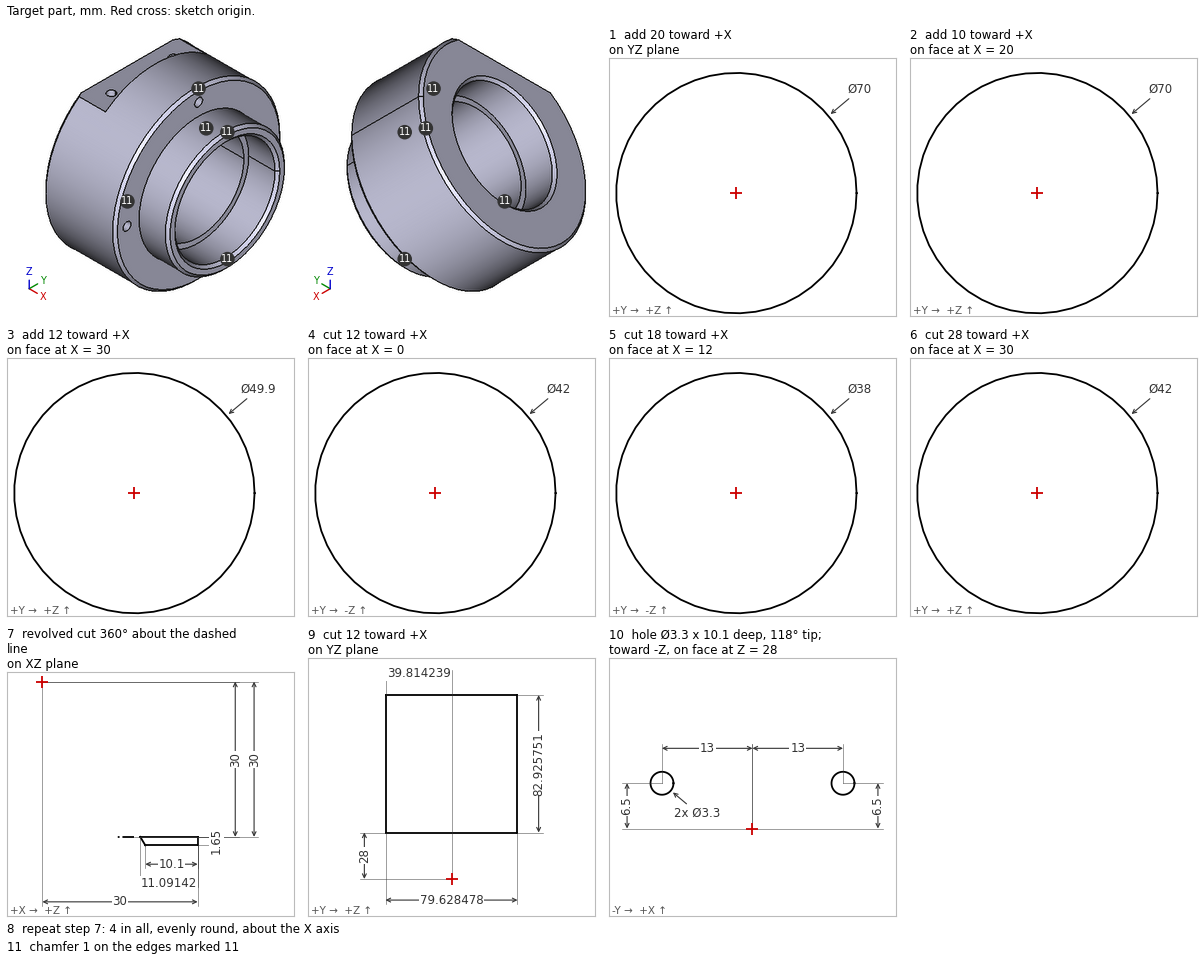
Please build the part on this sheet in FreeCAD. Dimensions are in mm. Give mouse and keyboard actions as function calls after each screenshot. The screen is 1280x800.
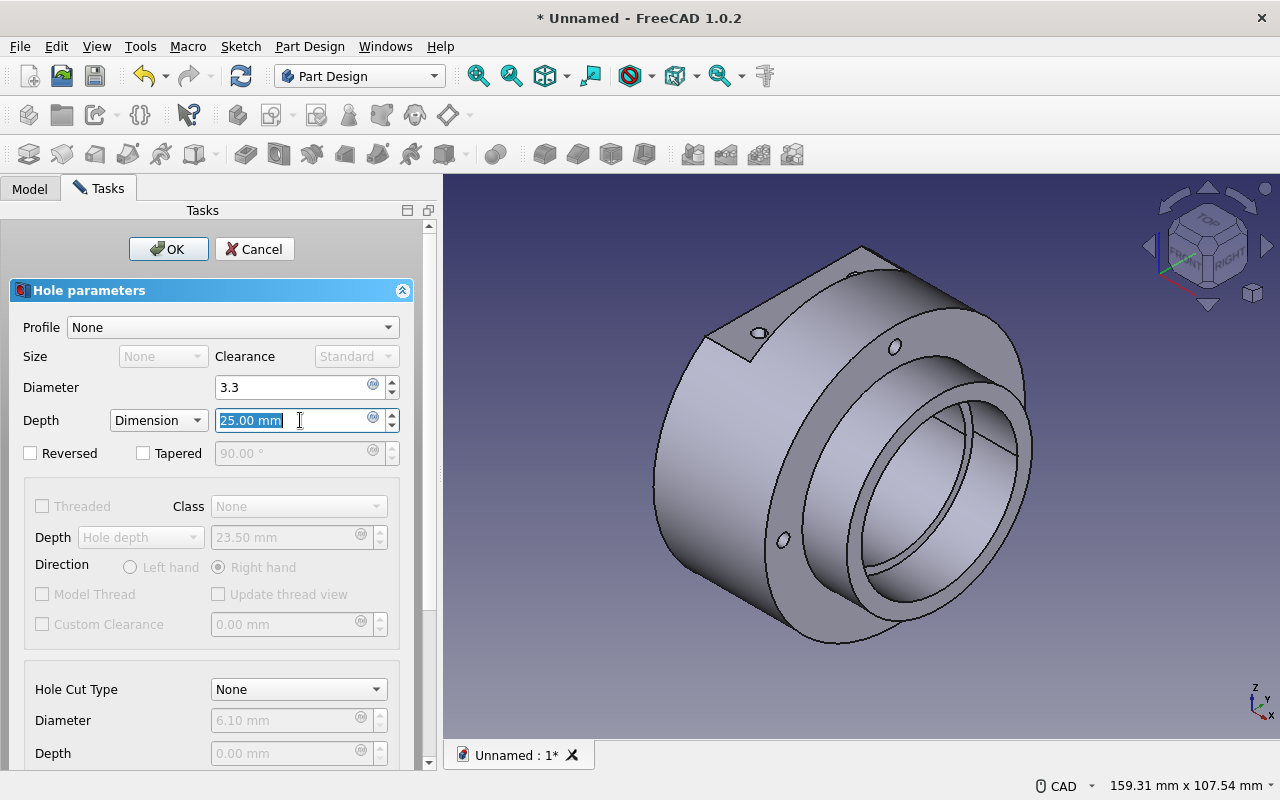
text(10.1)
key(Tab)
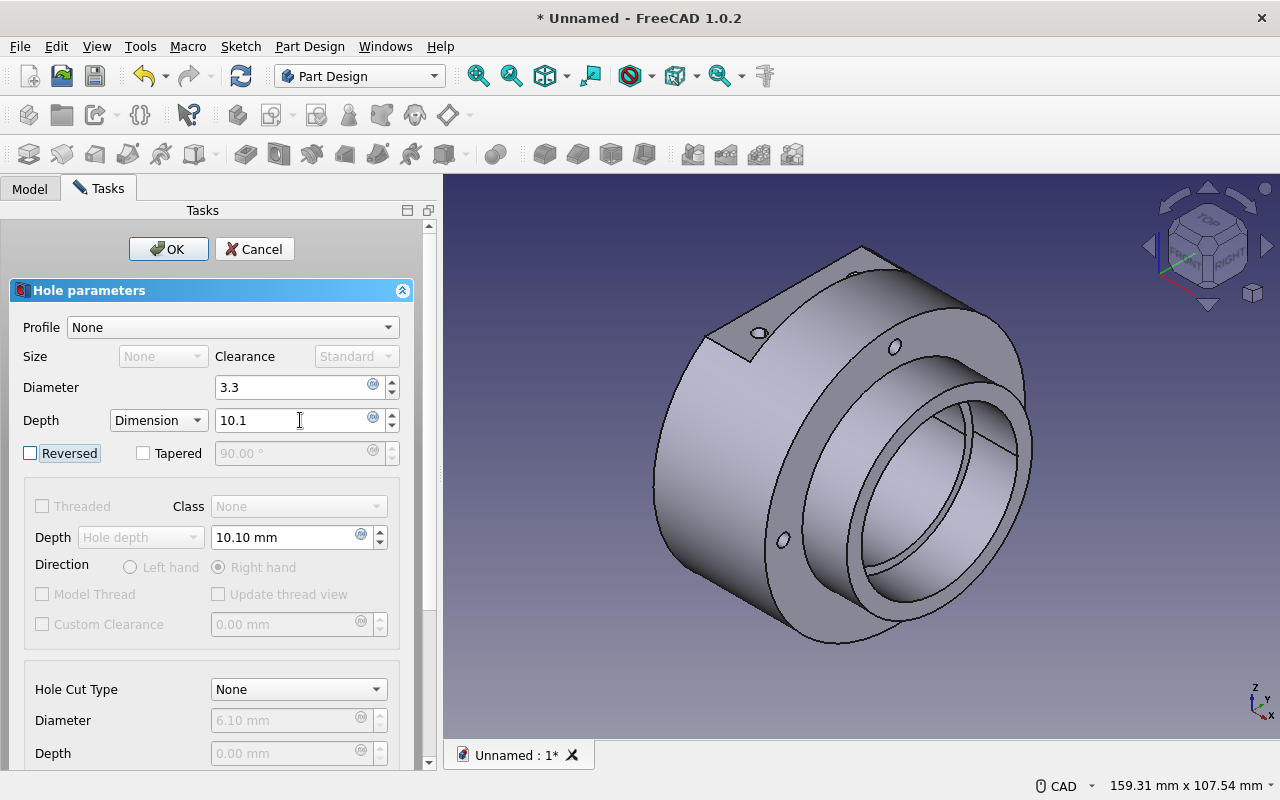
click(169, 249)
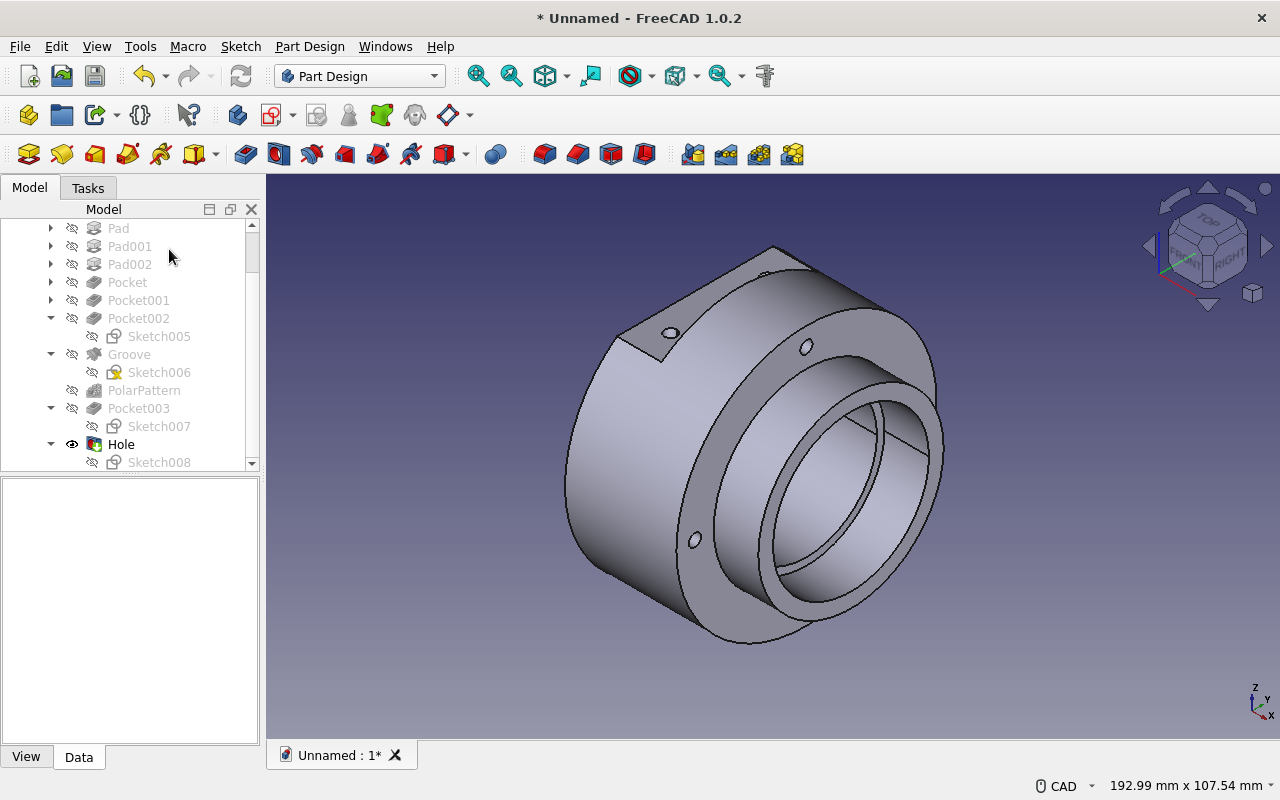
click(758, 554)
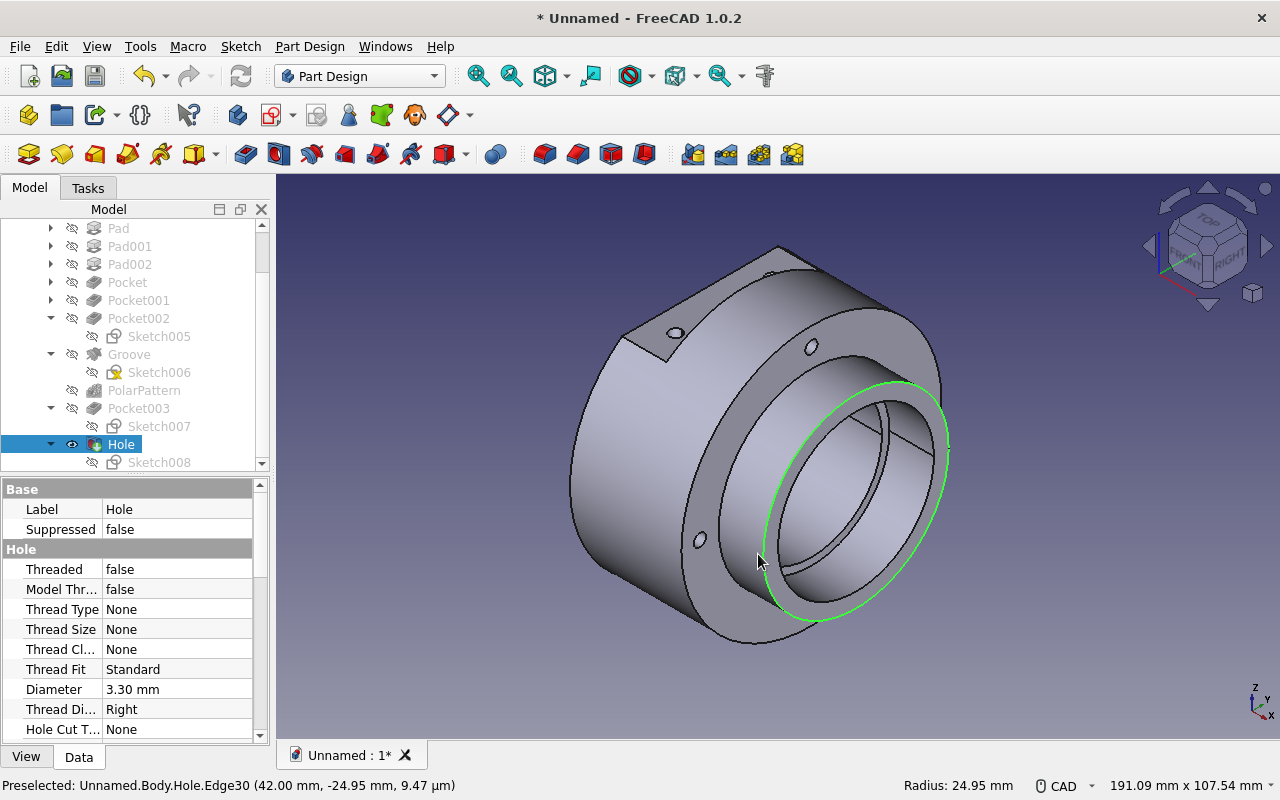
click(832, 600, ctrl)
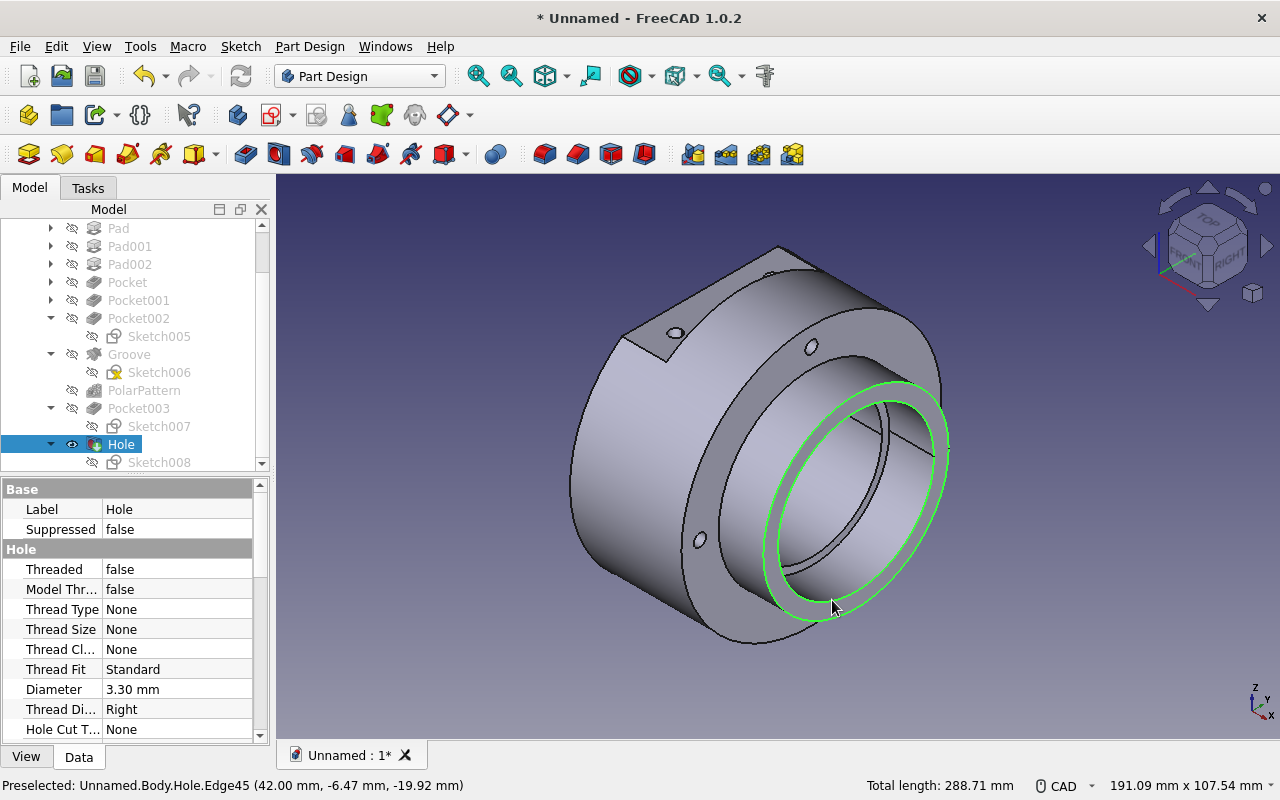
click(681, 550, ctrl)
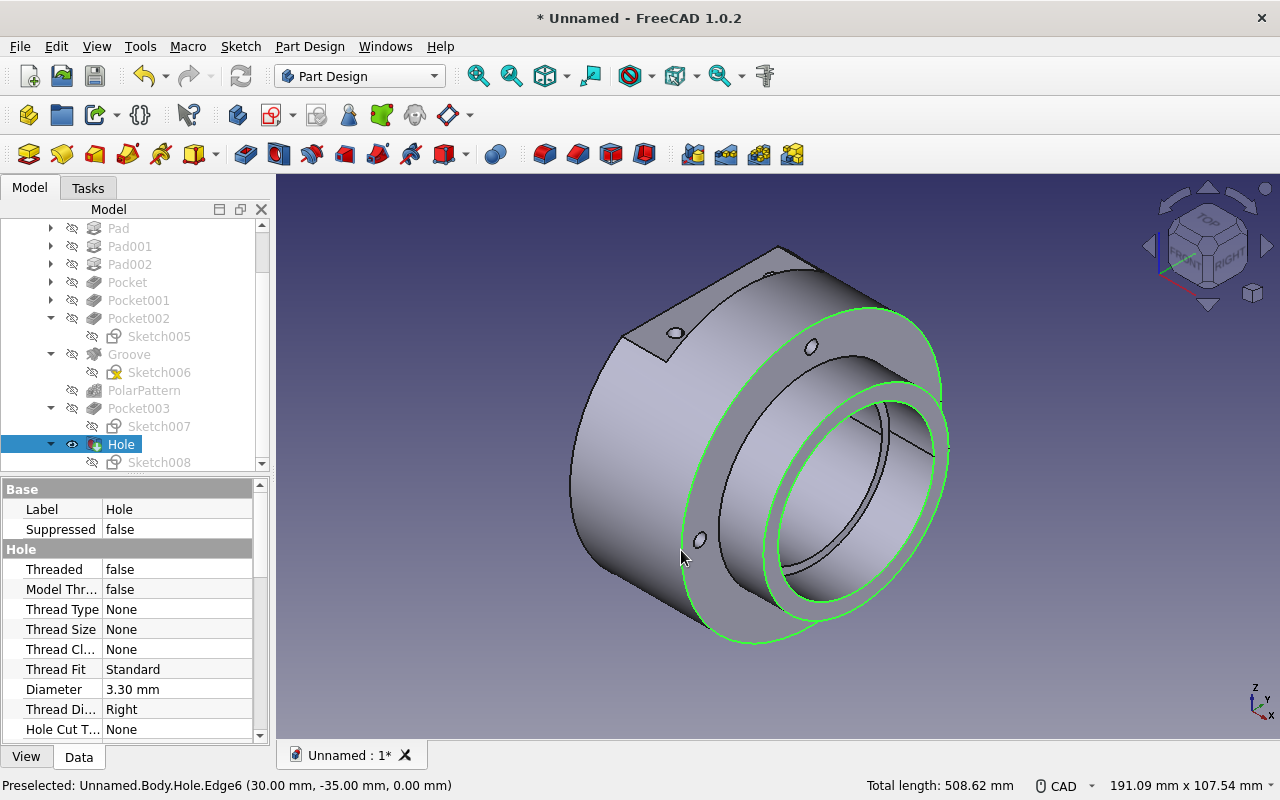
key(2)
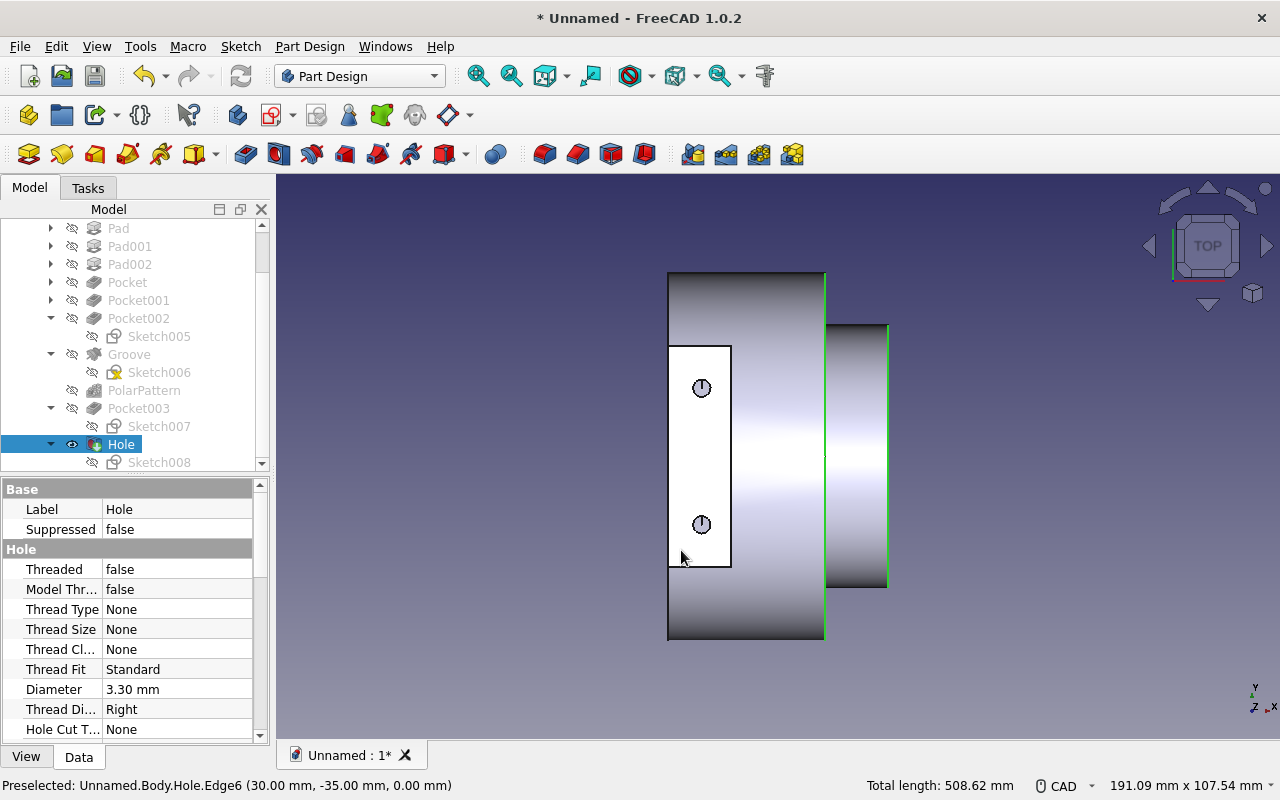
click(668, 583, ctrl)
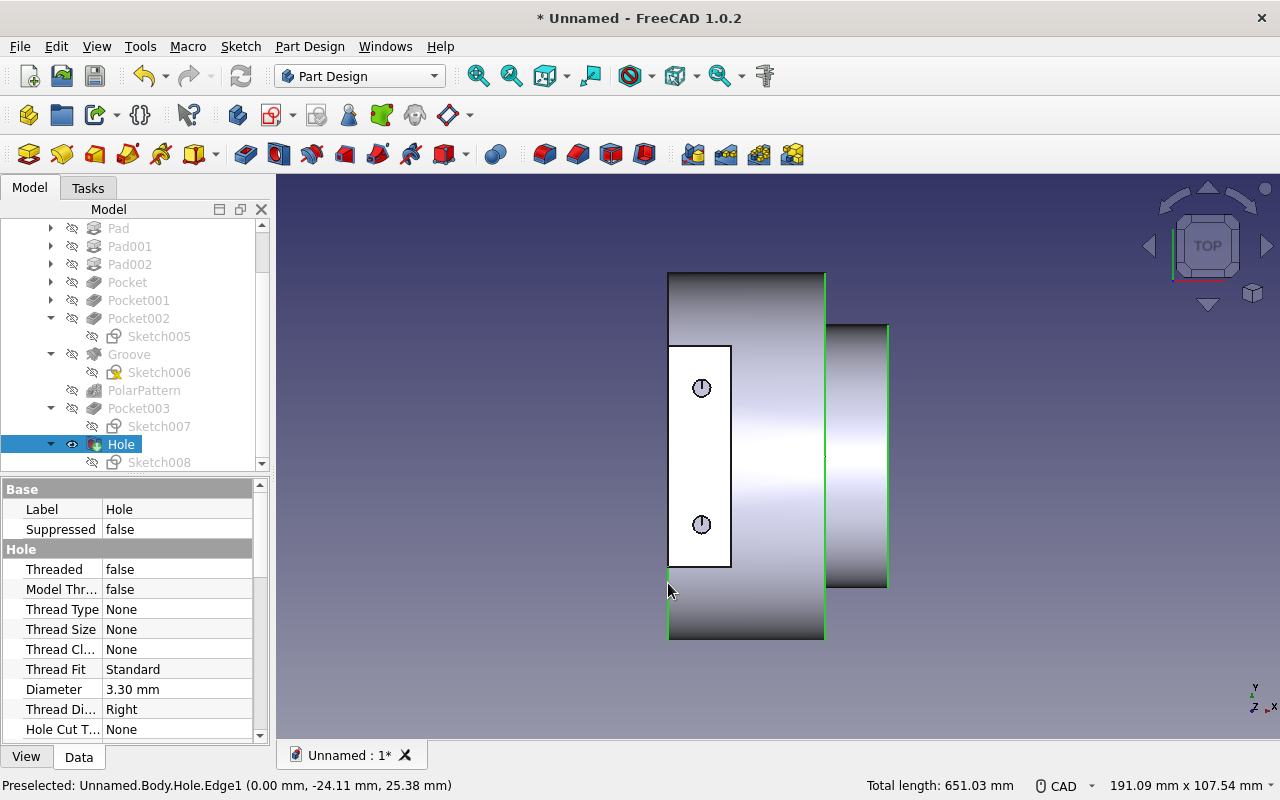
key(0)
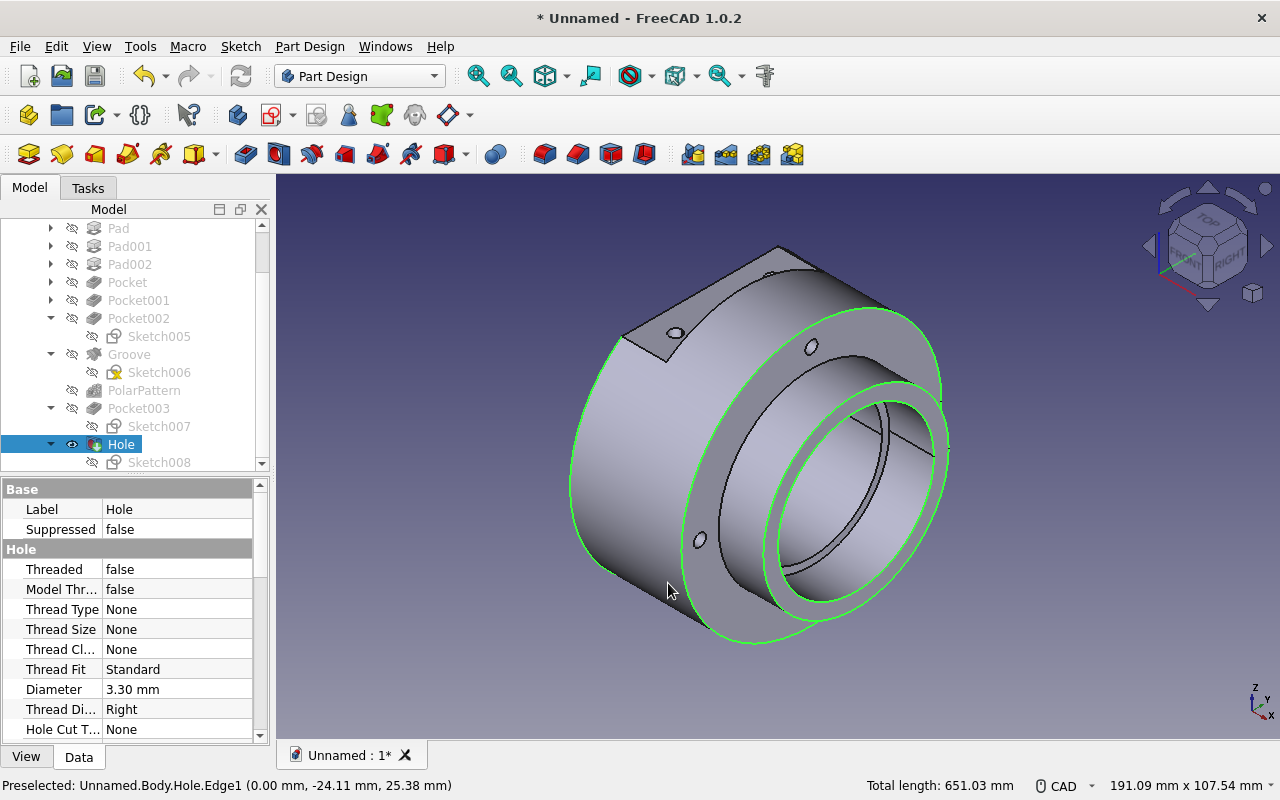
key(1)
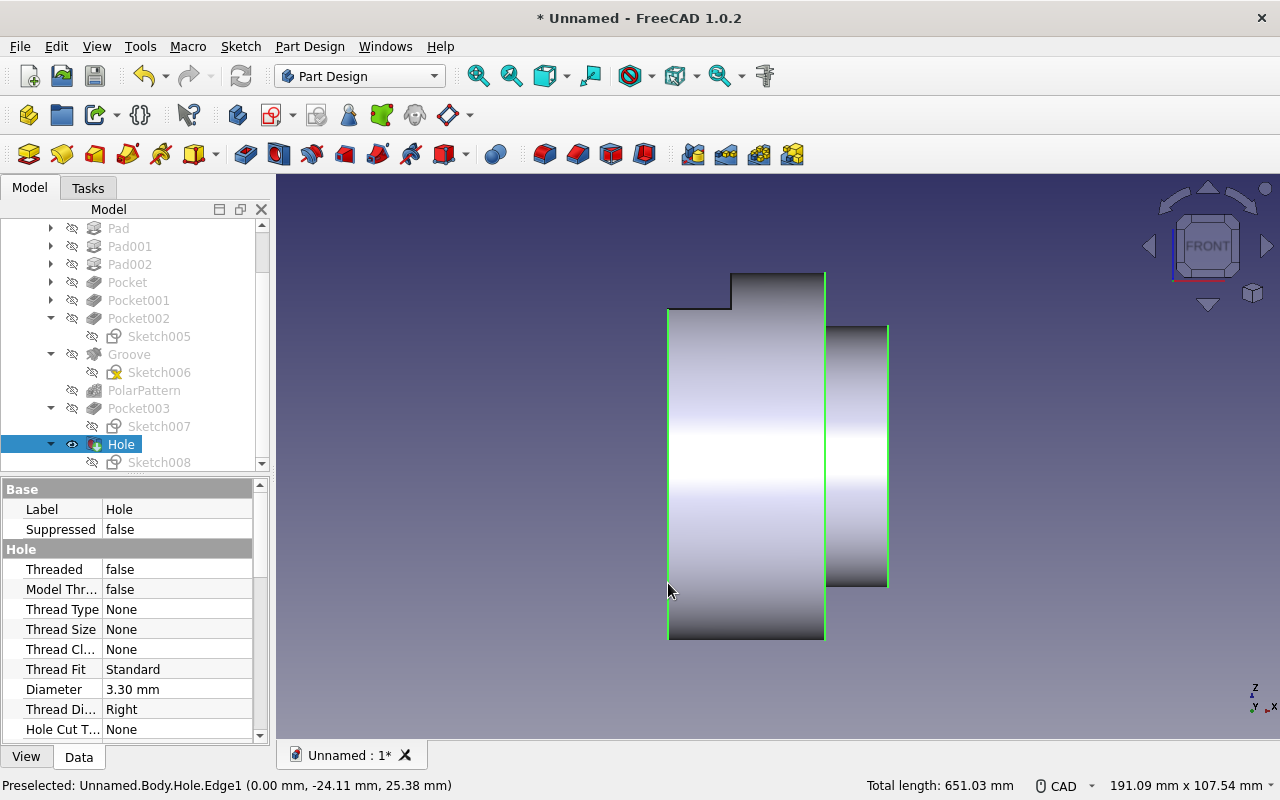
key(3)